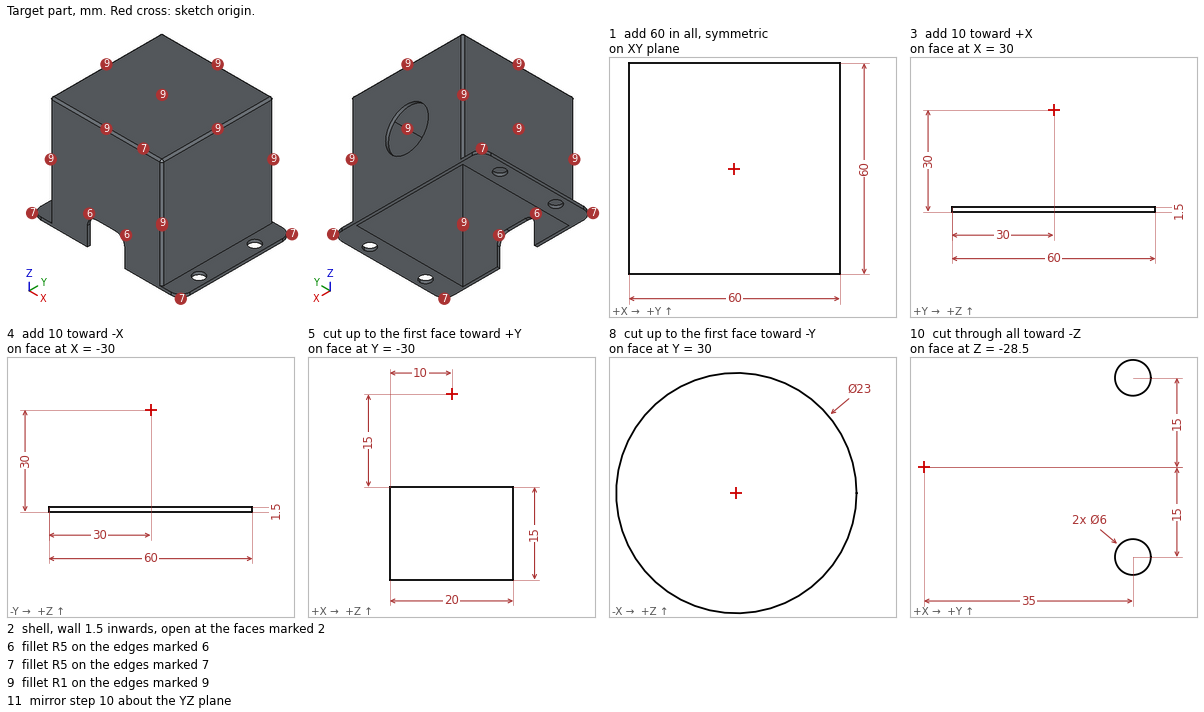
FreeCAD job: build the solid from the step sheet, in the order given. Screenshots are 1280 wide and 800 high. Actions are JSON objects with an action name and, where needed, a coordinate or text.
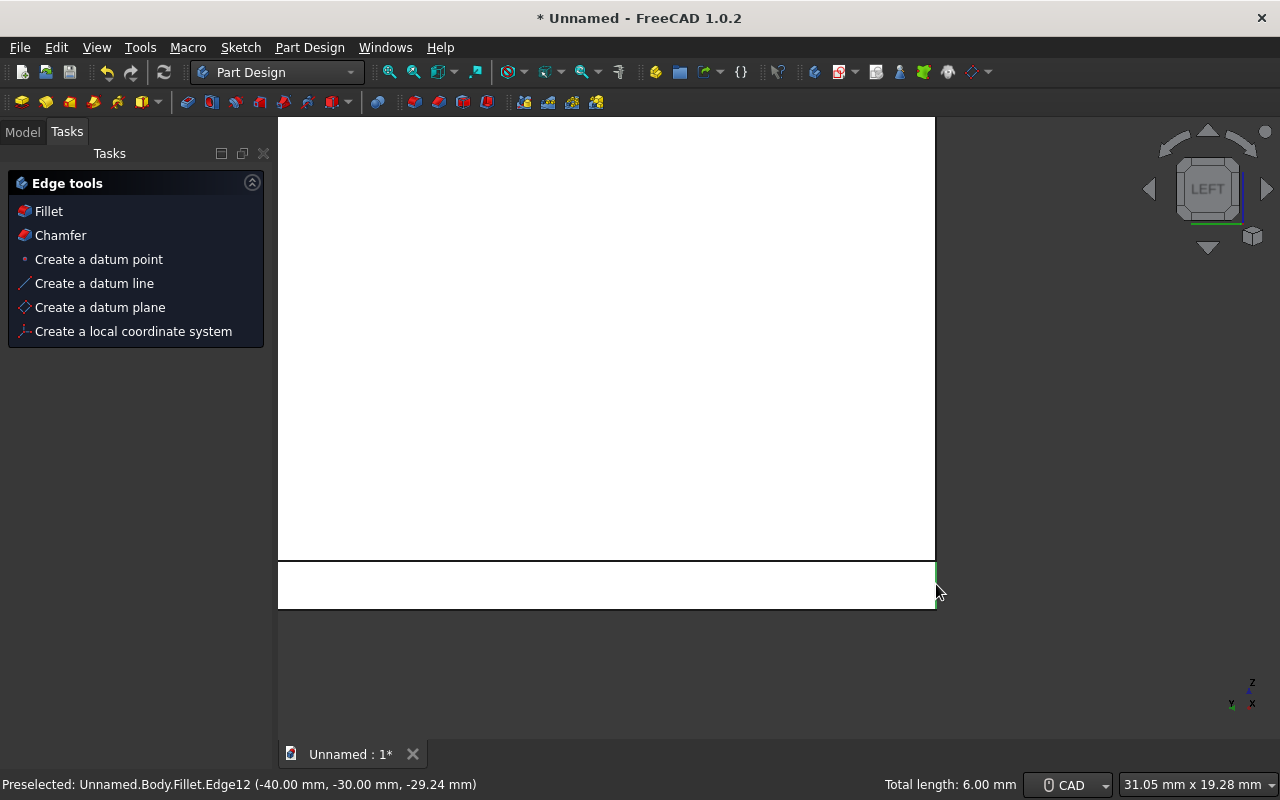
{"action": "left_click", "coordinate": [416, 102]}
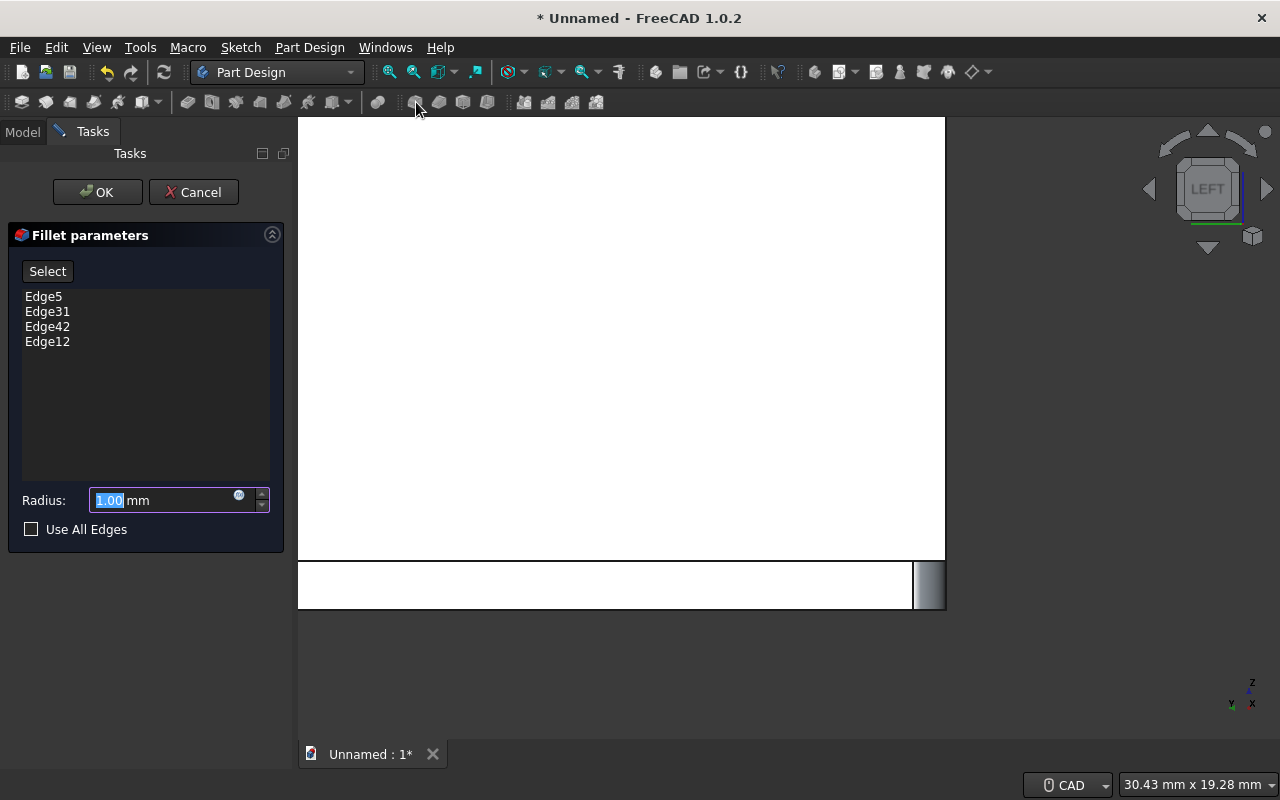
{"action": "type", "text": "5"}
{"action": "key", "text": "Tab"}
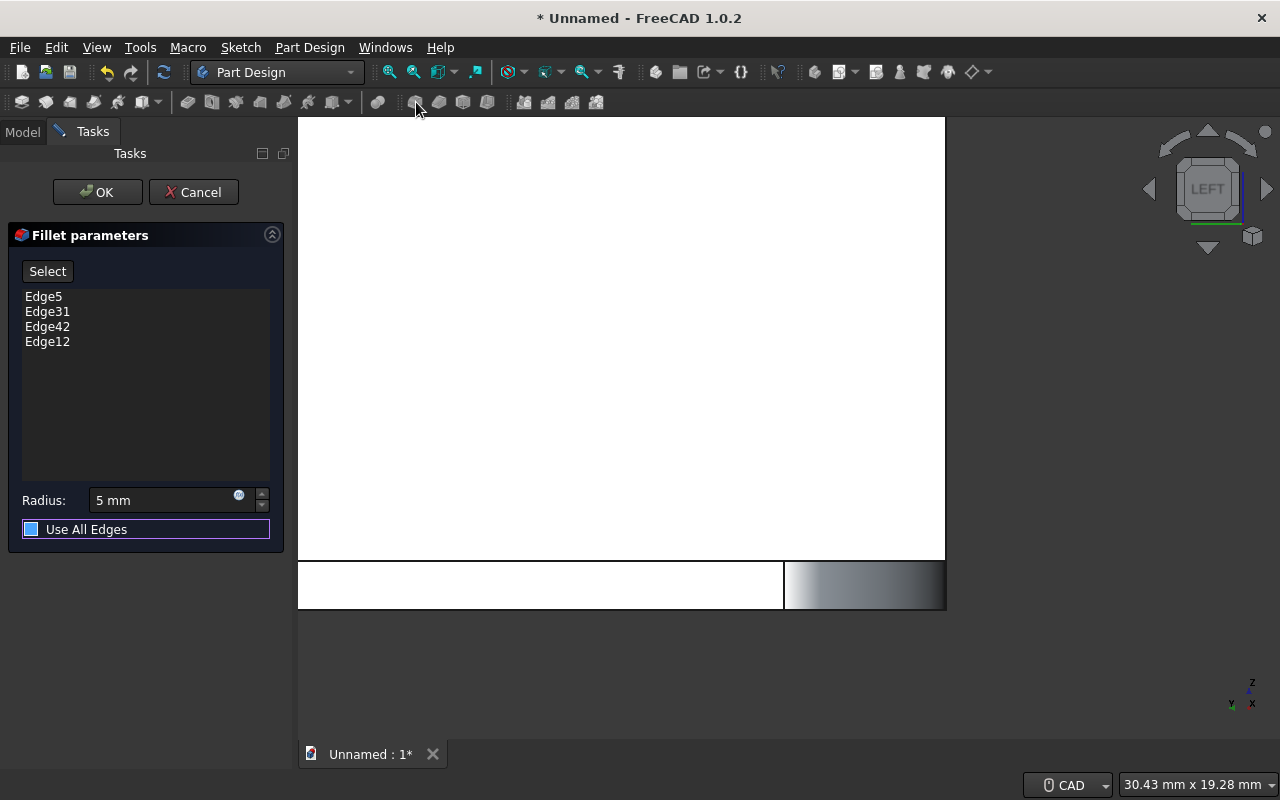
{"action": "left_click", "coordinate": [98, 192]}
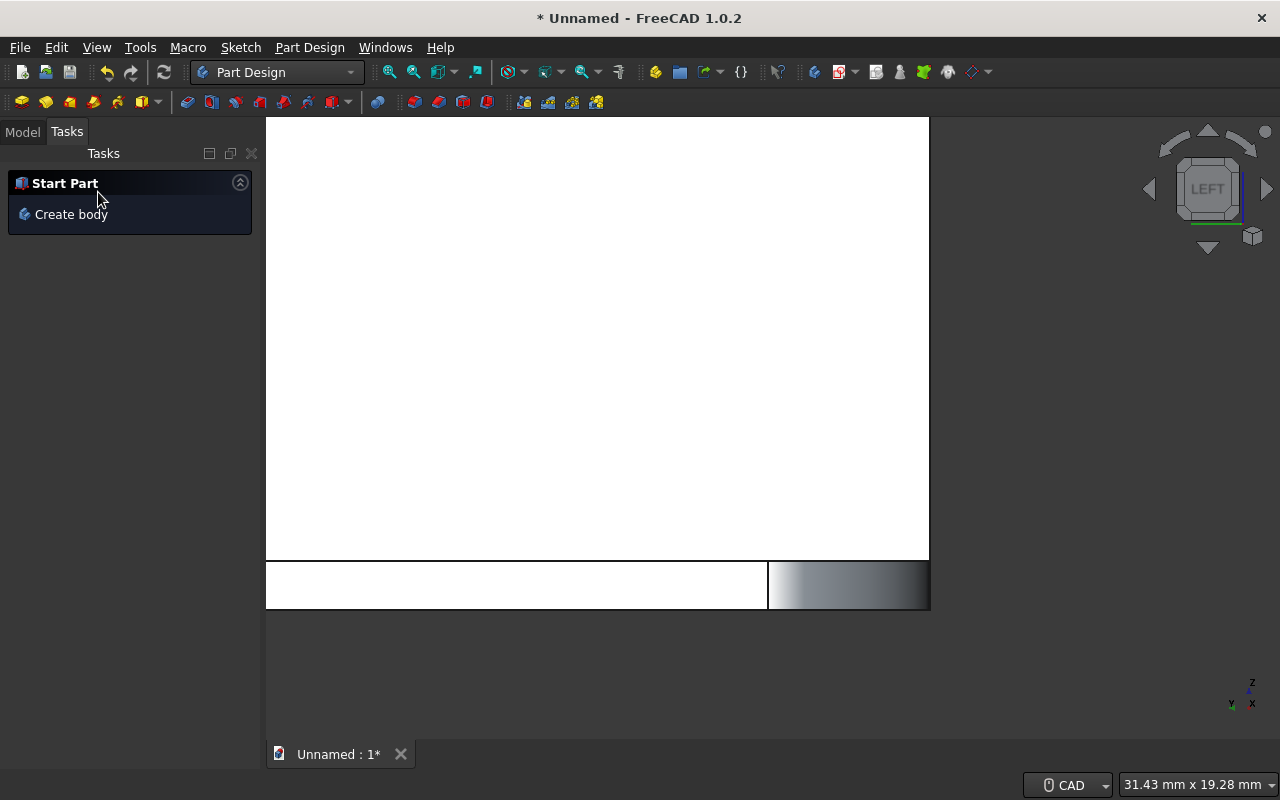
{"action": "left_click", "coordinate": [390, 72]}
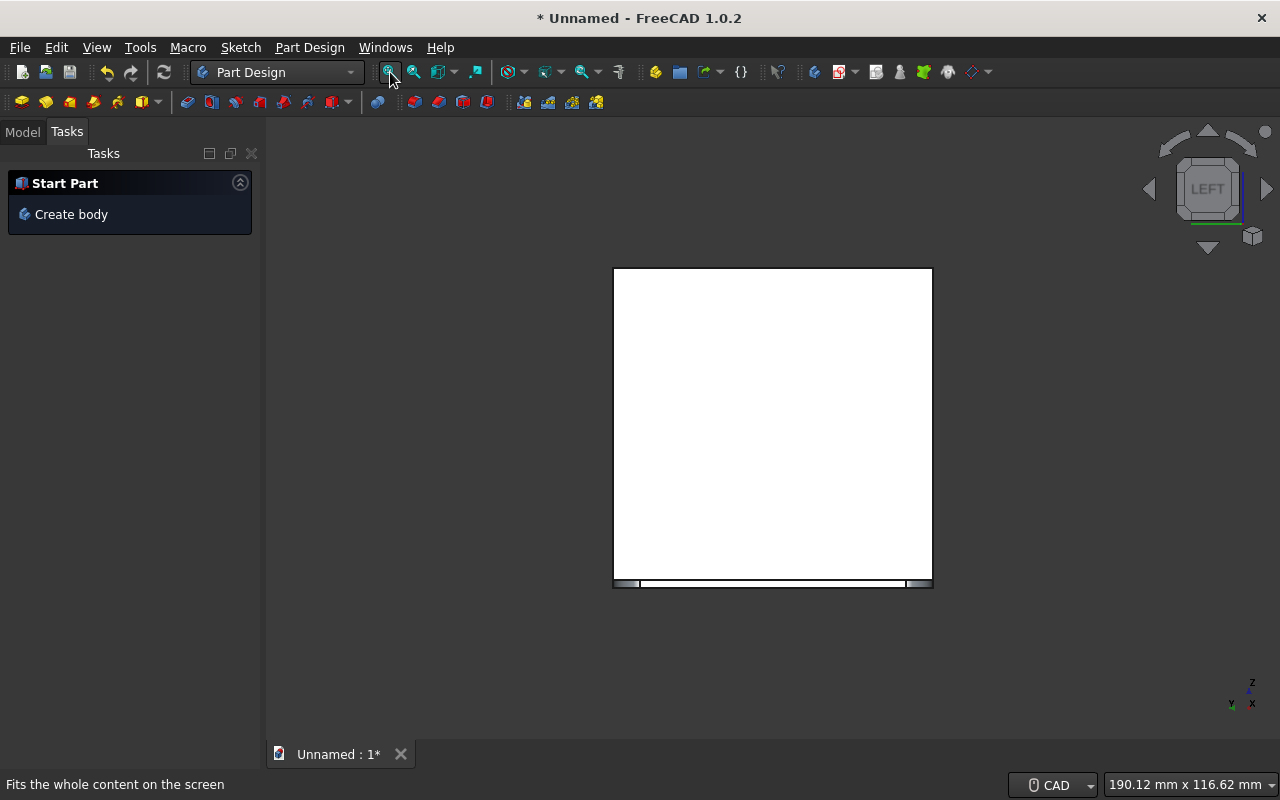
{"action": "key", "text": "4"}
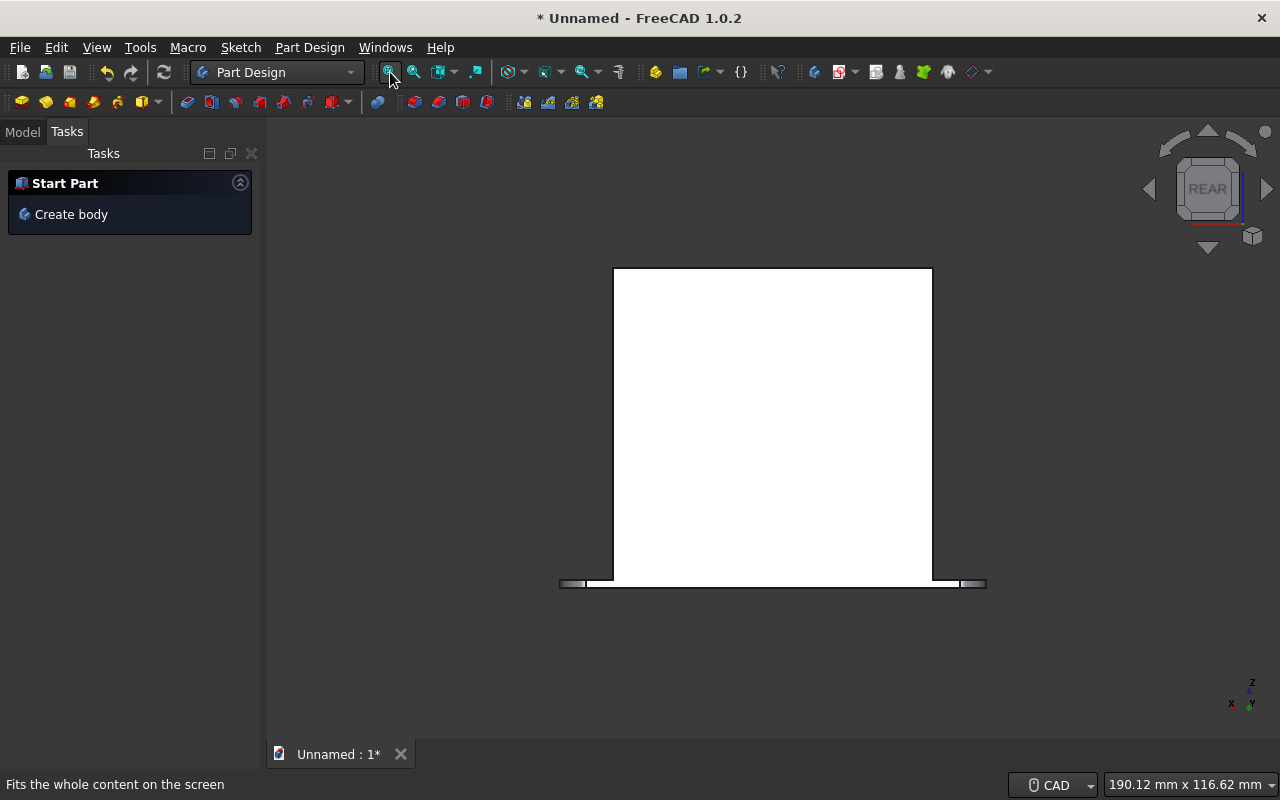
{"action": "left_click", "coordinate": [773, 427]}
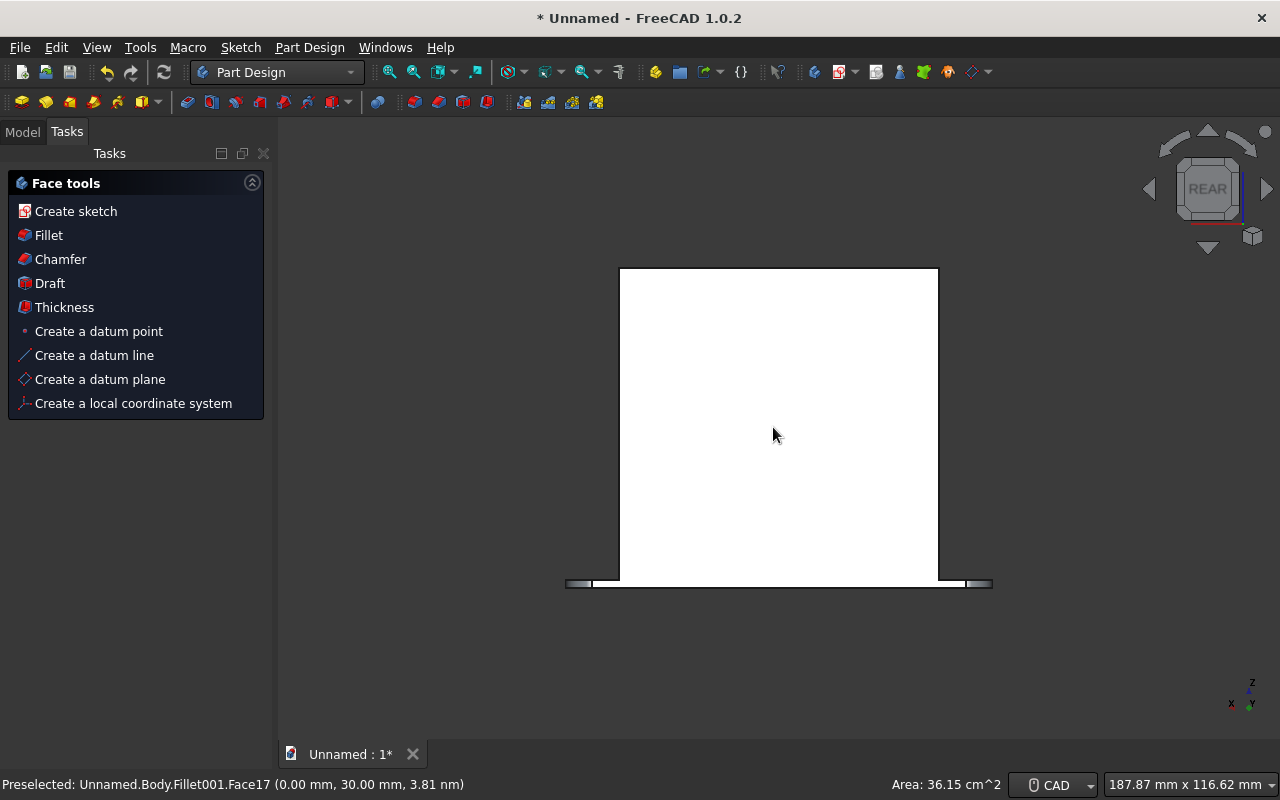
{"action": "left_click", "coordinate": [840, 72]}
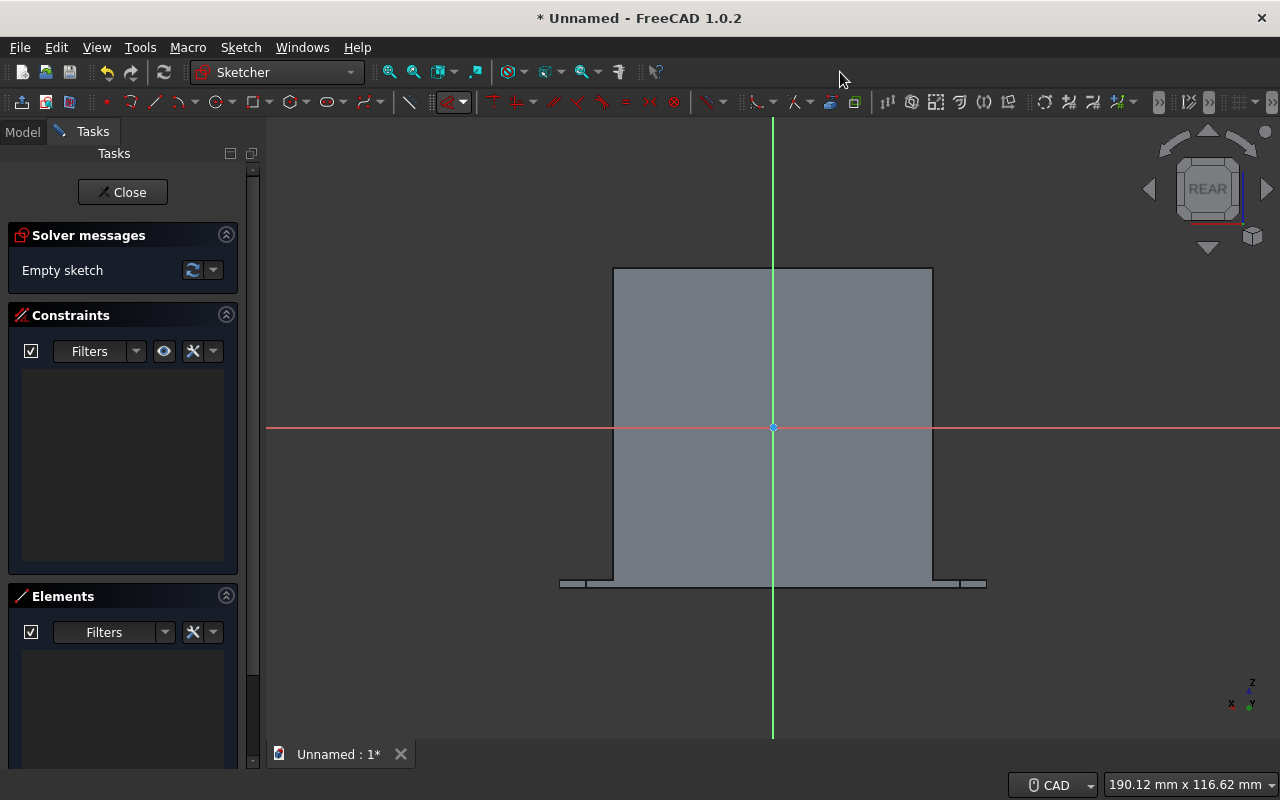
{"action": "scroll", "coordinate": [803, 428], "scroll_direction": "up", "scroll_amount": 6}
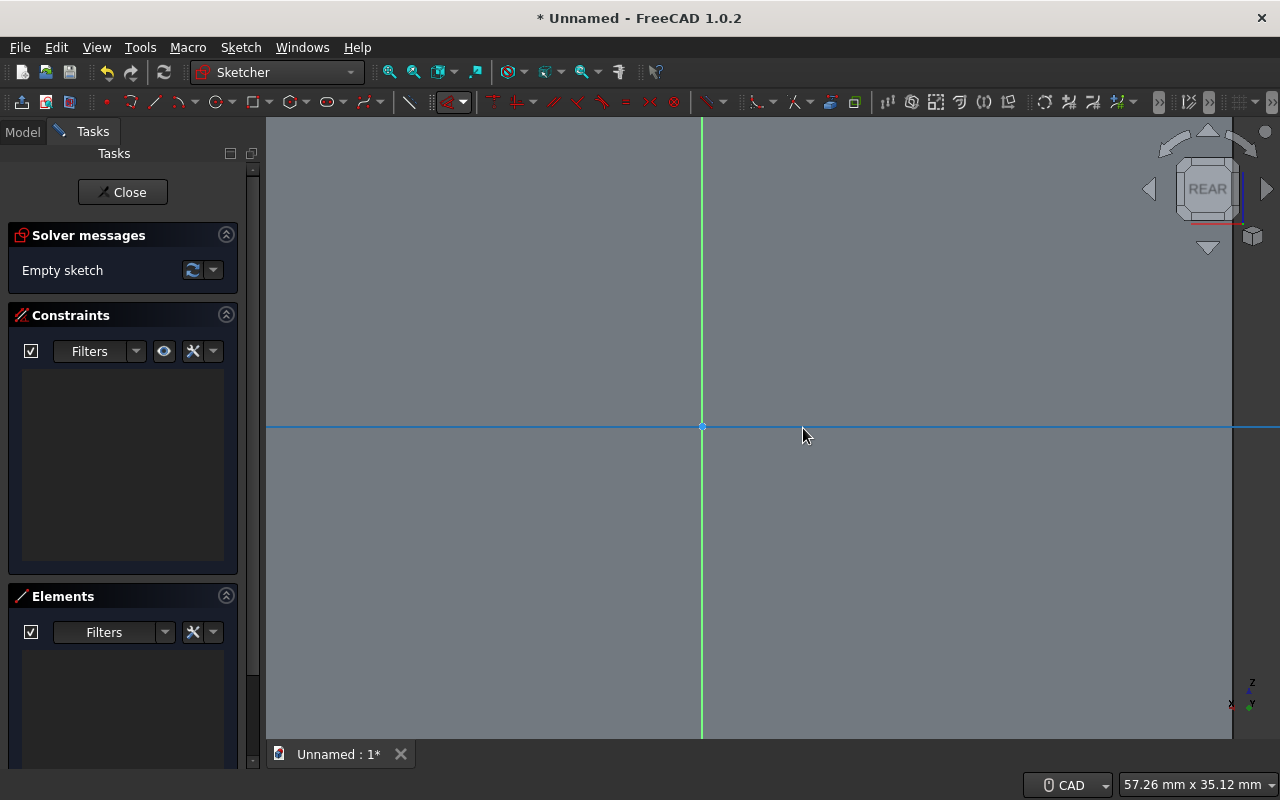
{"action": "key", "text": "g c"}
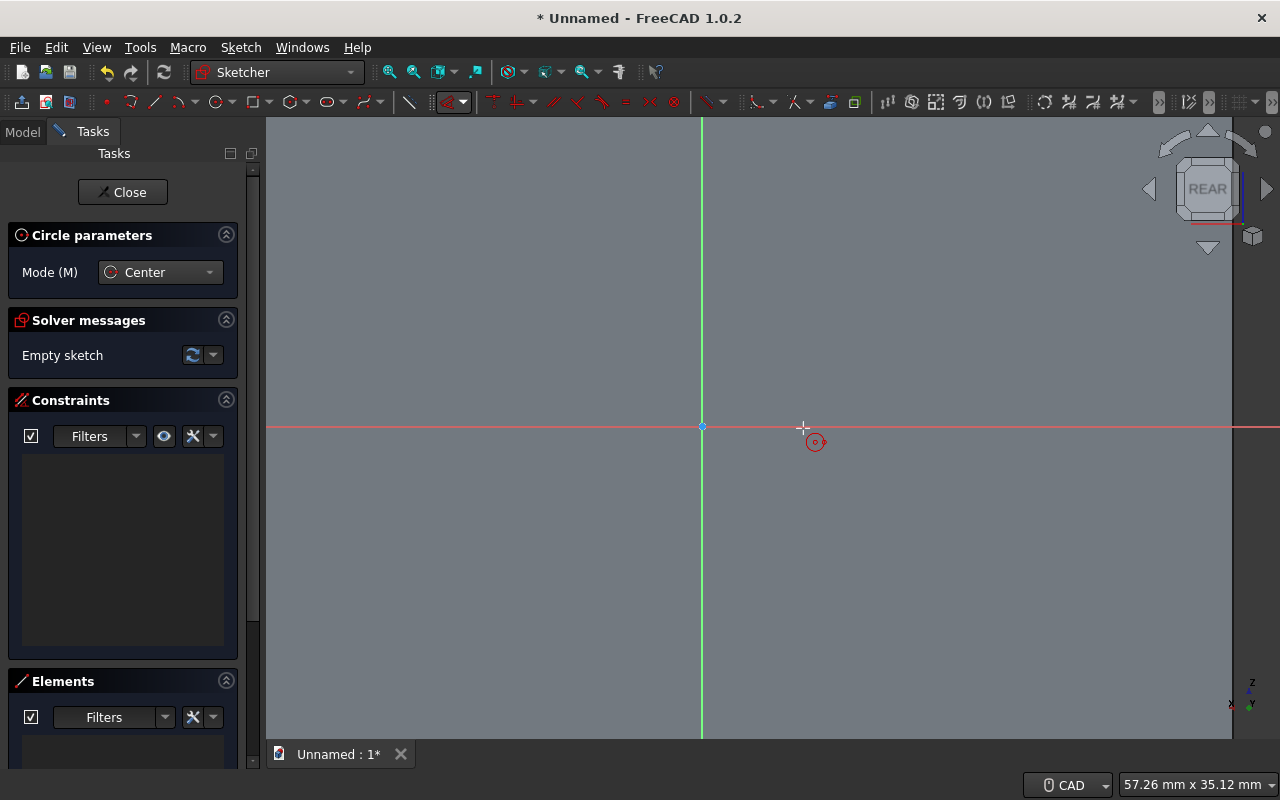
{"action": "left_click", "coordinate": [702, 427]}
{"action": "mouse_move", "coordinate": [846, 283]}